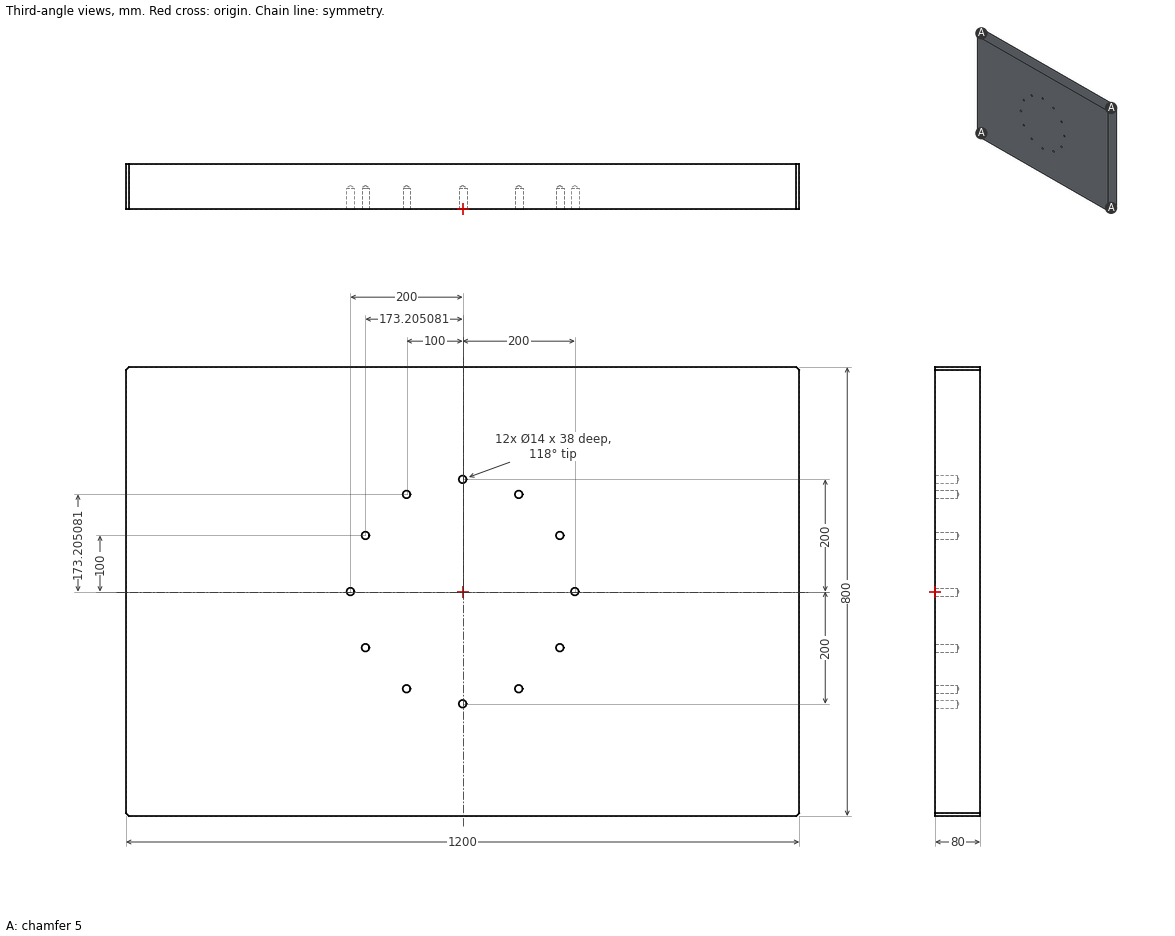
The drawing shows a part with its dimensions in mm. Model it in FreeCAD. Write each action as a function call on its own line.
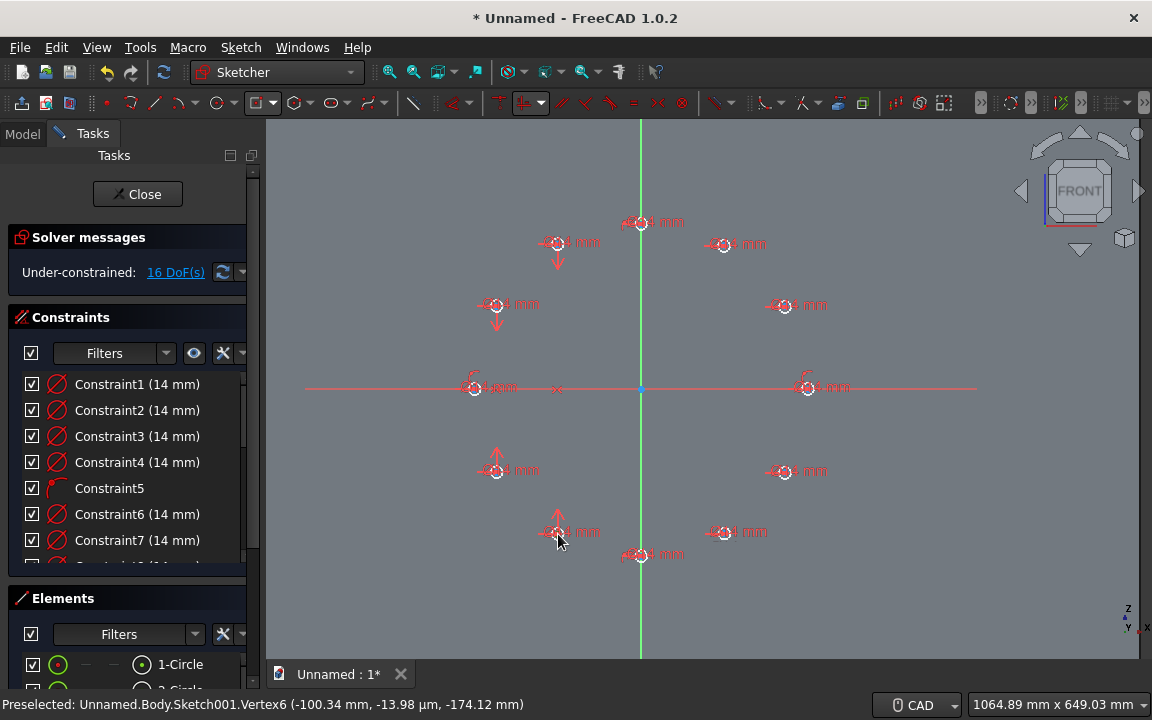
click(724, 534)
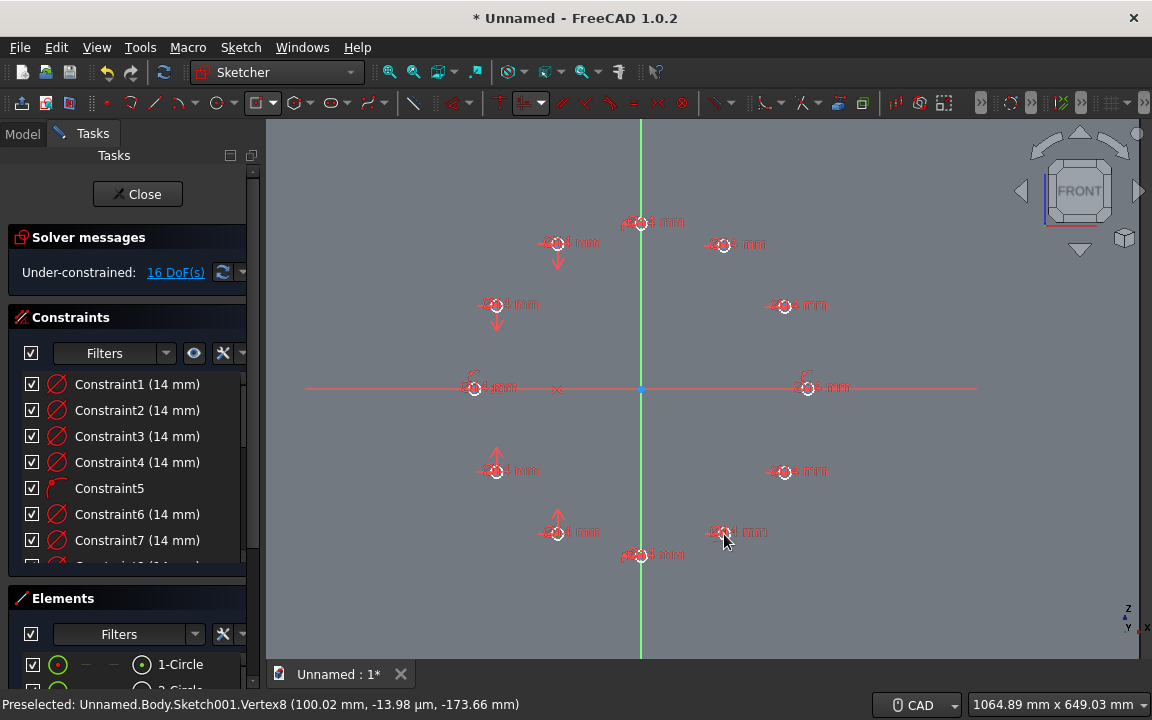
click(641, 596)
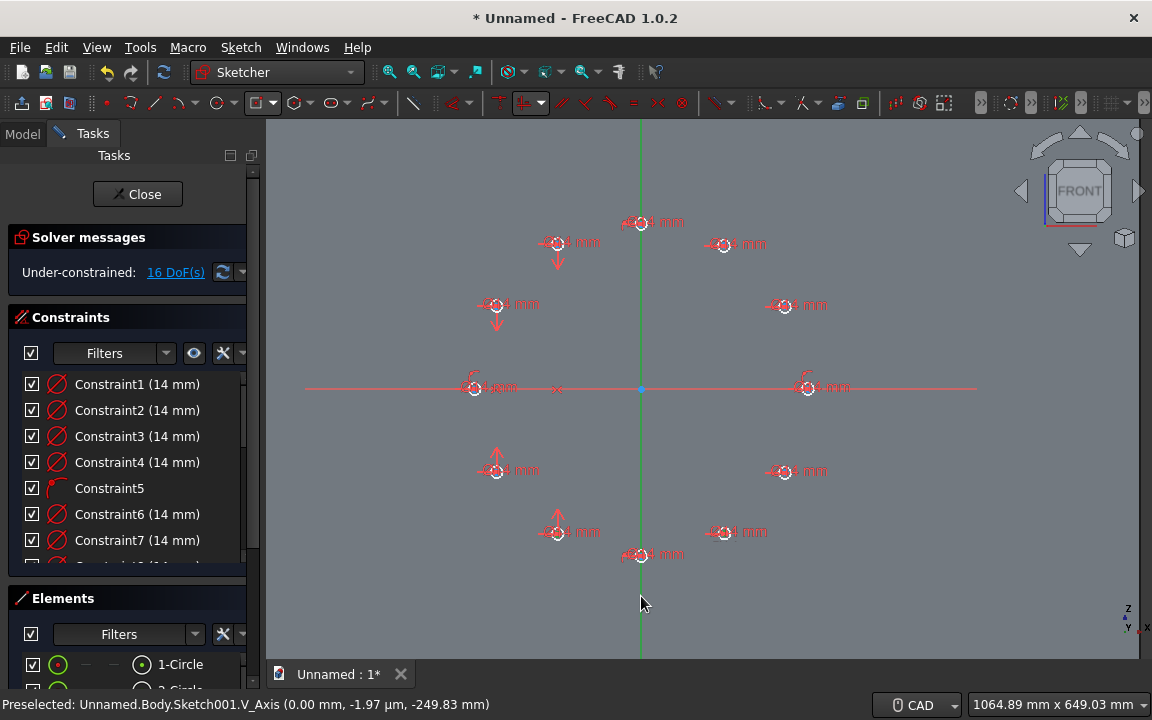
click(658, 104)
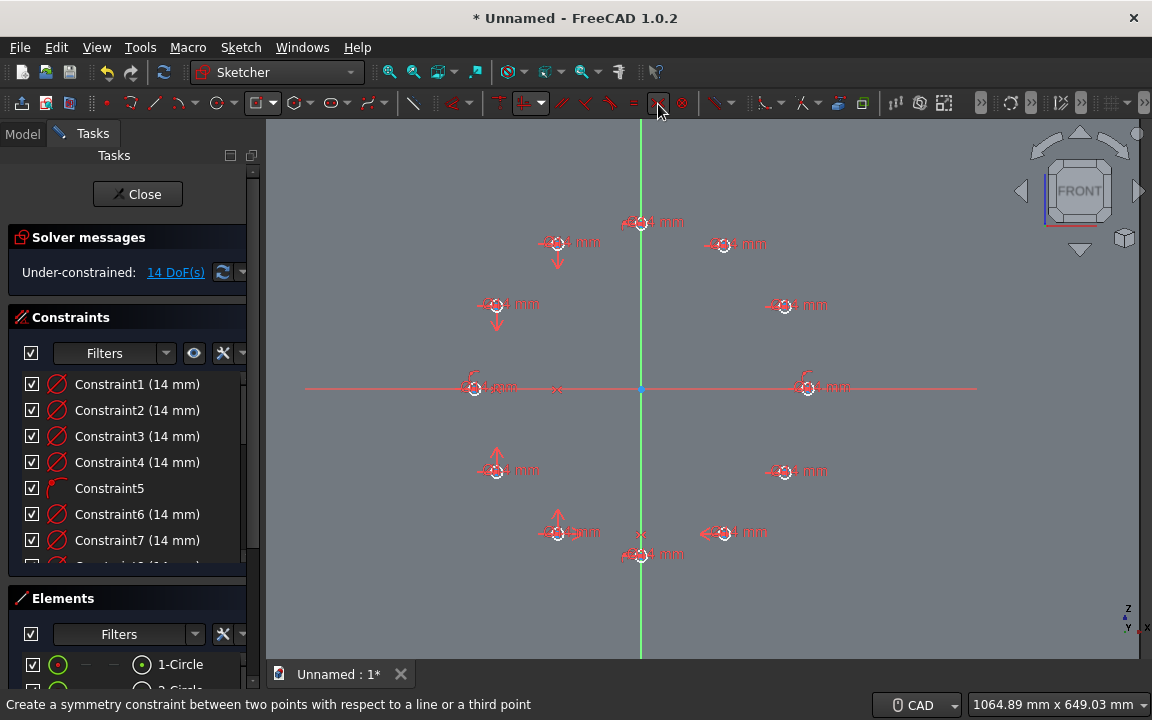
click(497, 472)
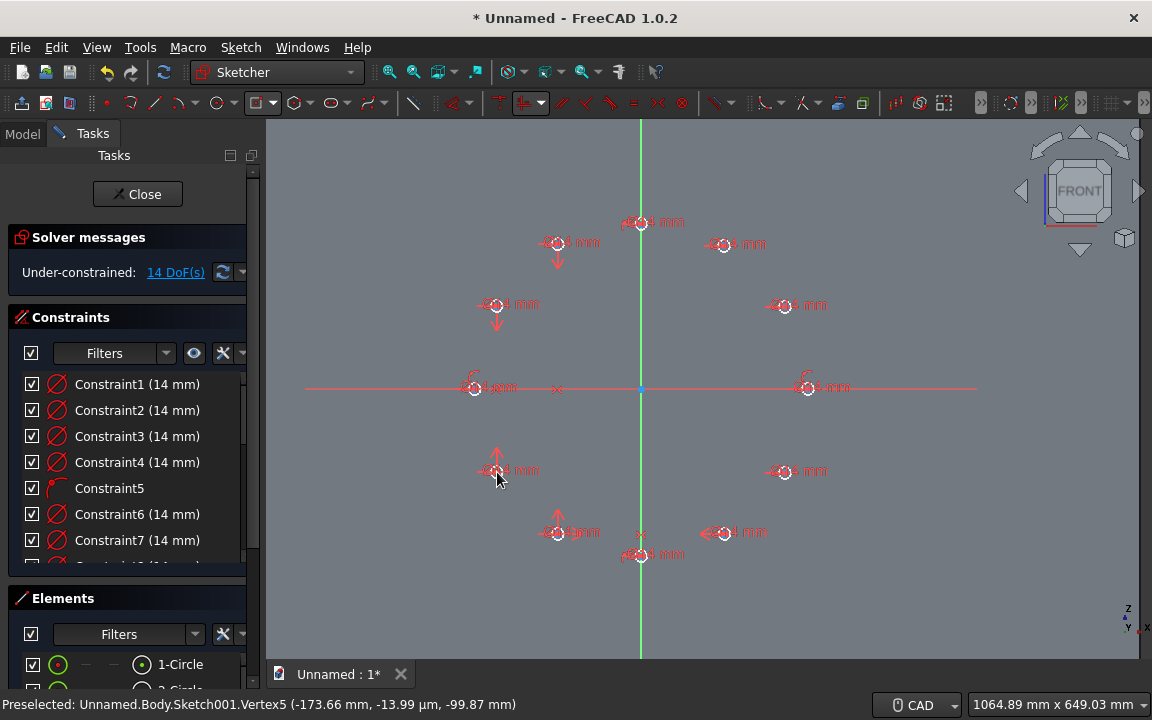
click(785, 473)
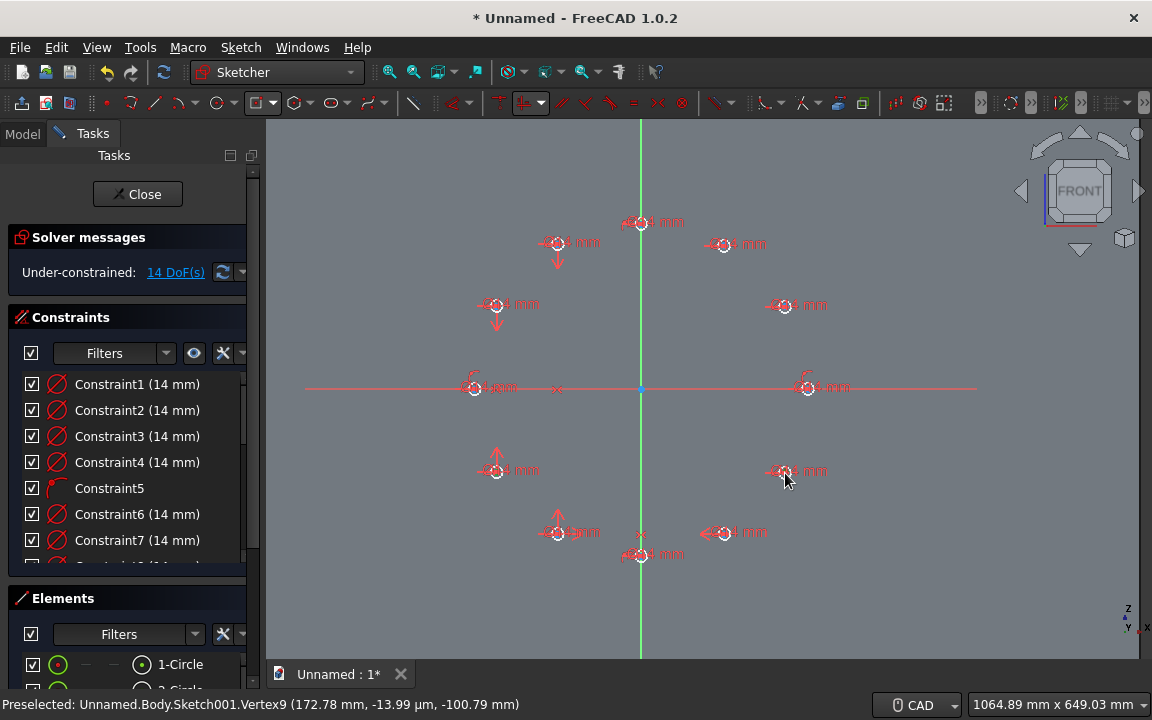
click(641, 596)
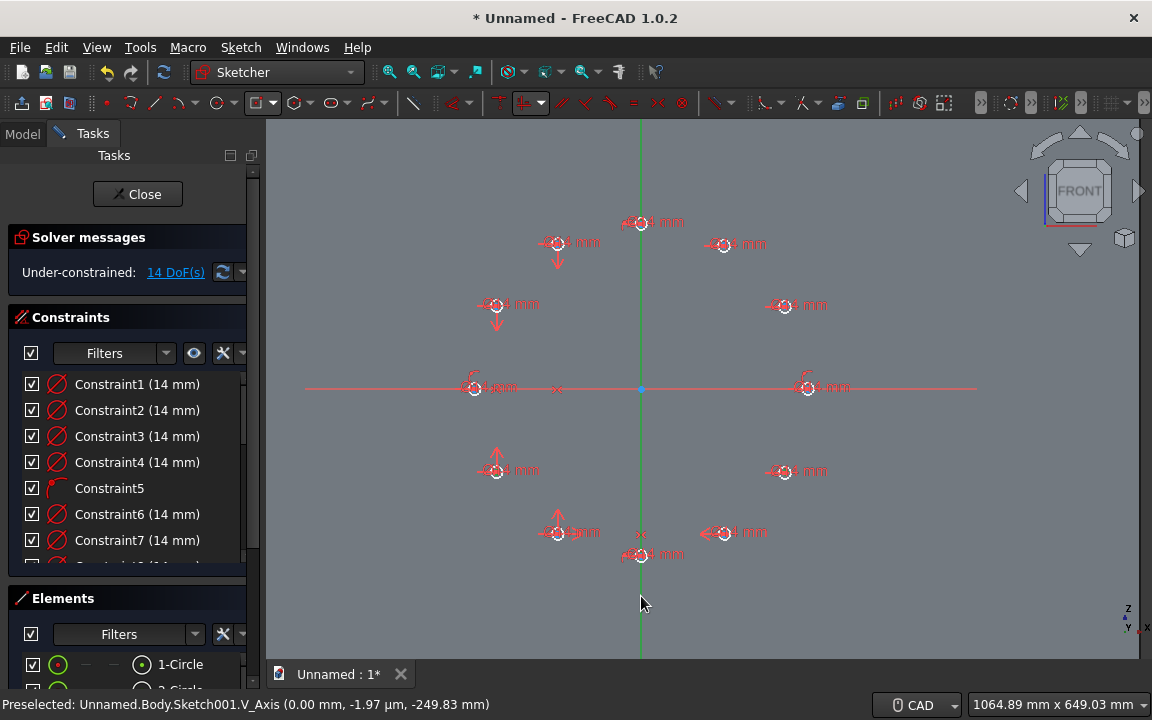
click(658, 104)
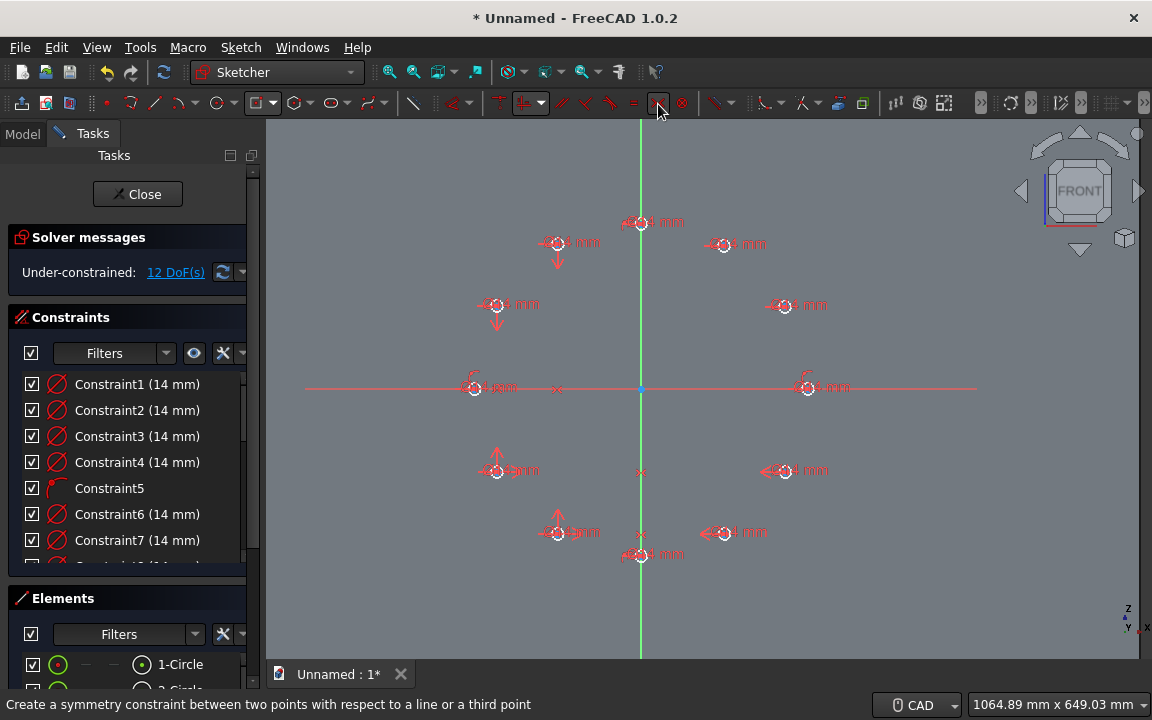
click(497, 306)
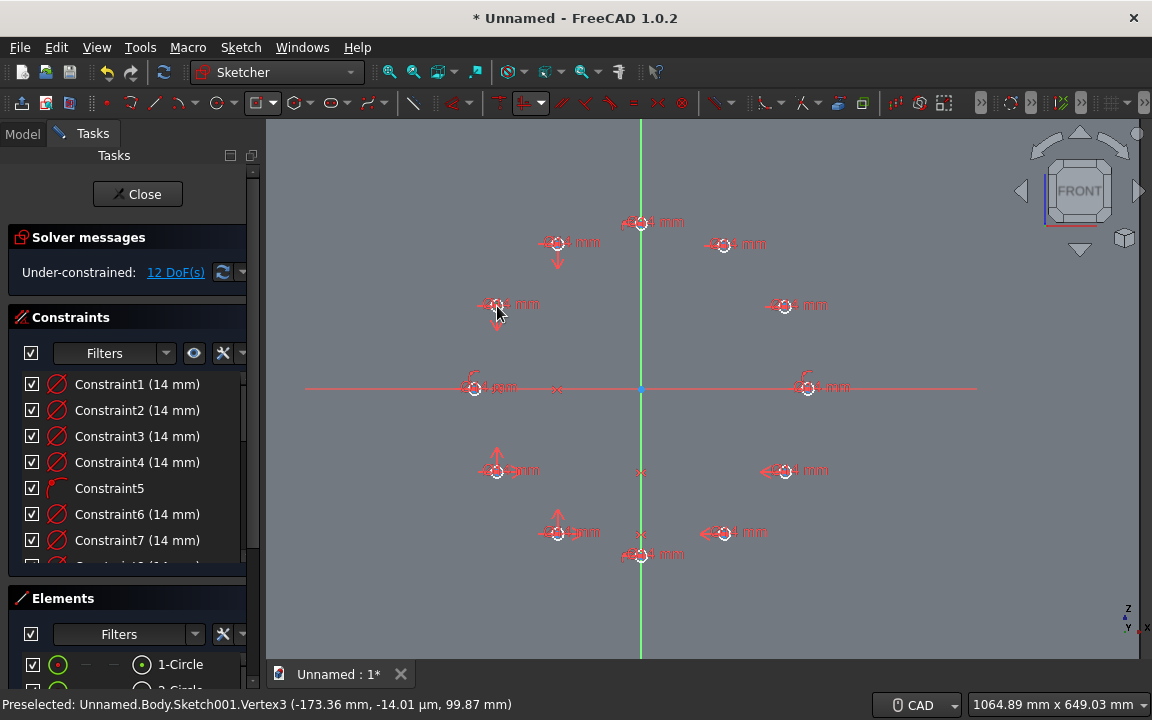
click(785, 307)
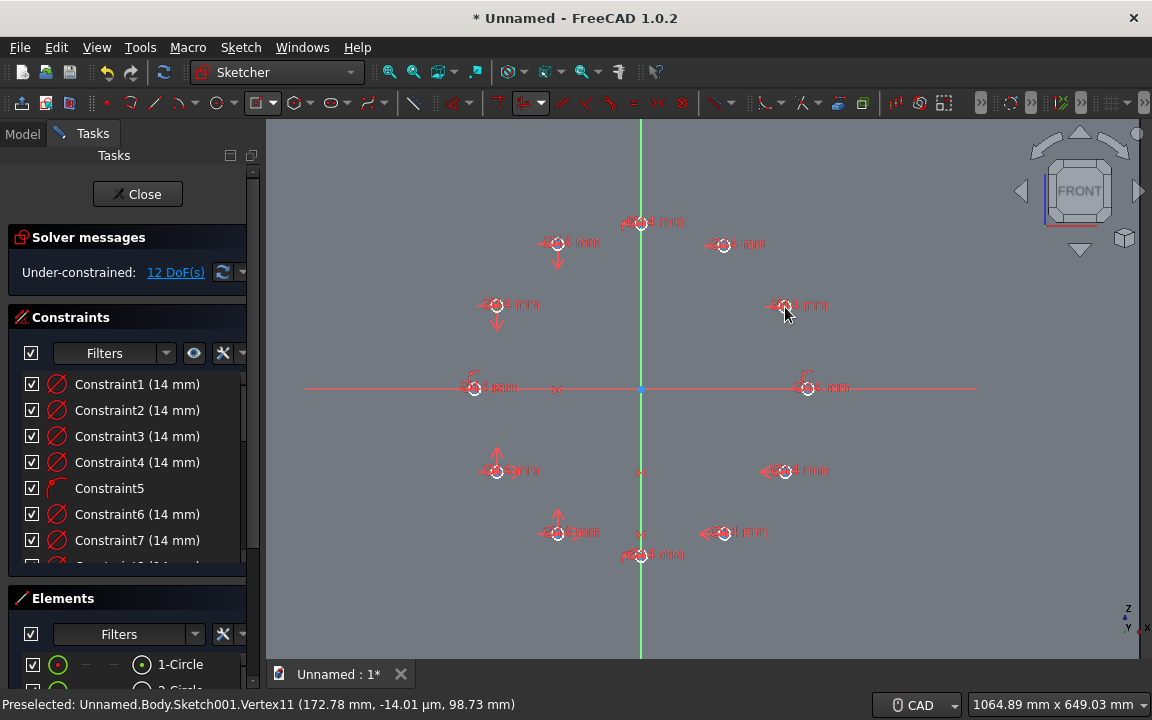
click(641, 596)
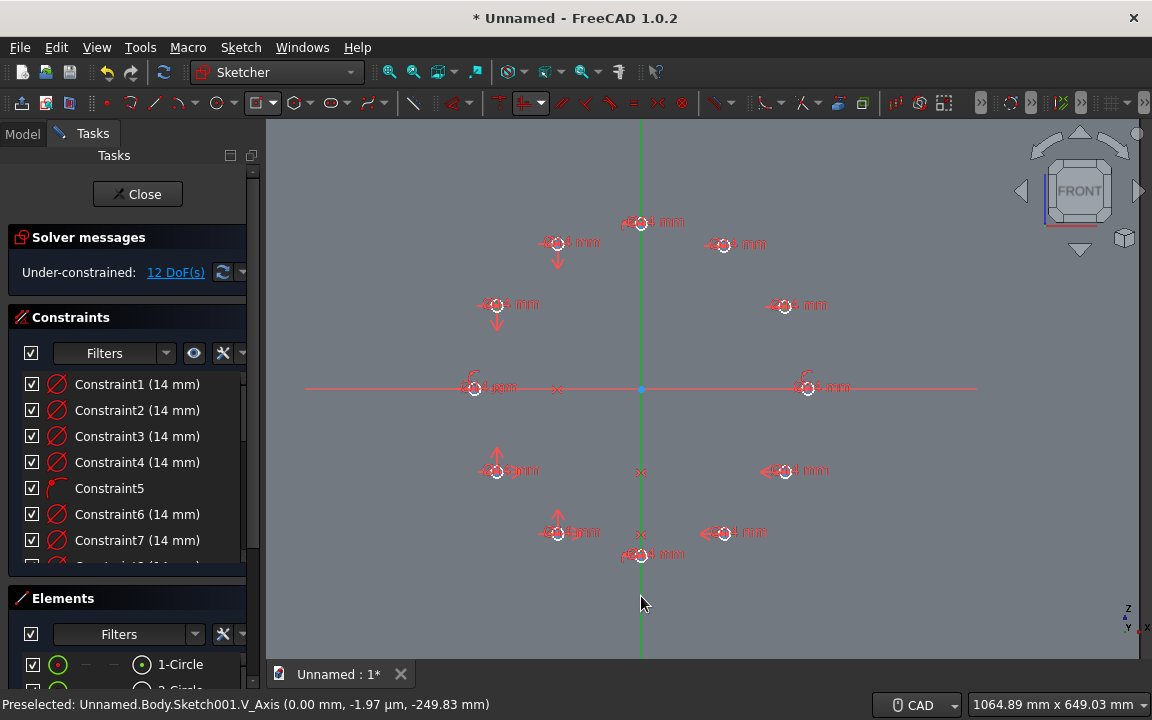
click(658, 104)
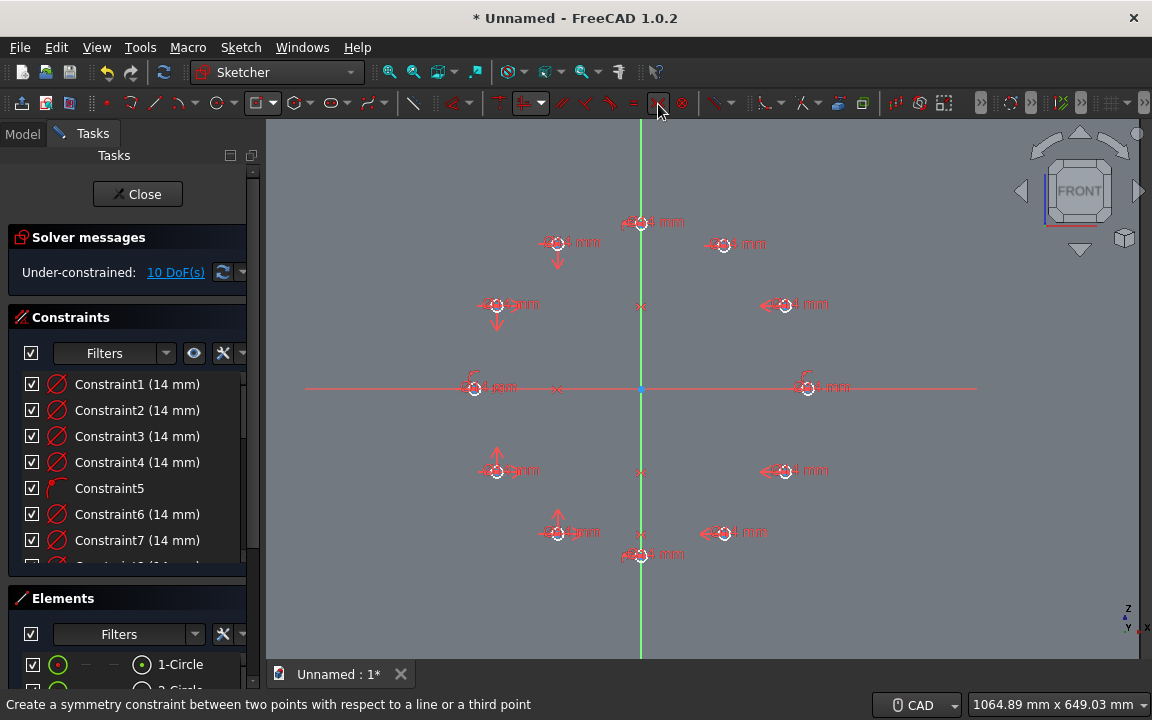
click(558, 244)